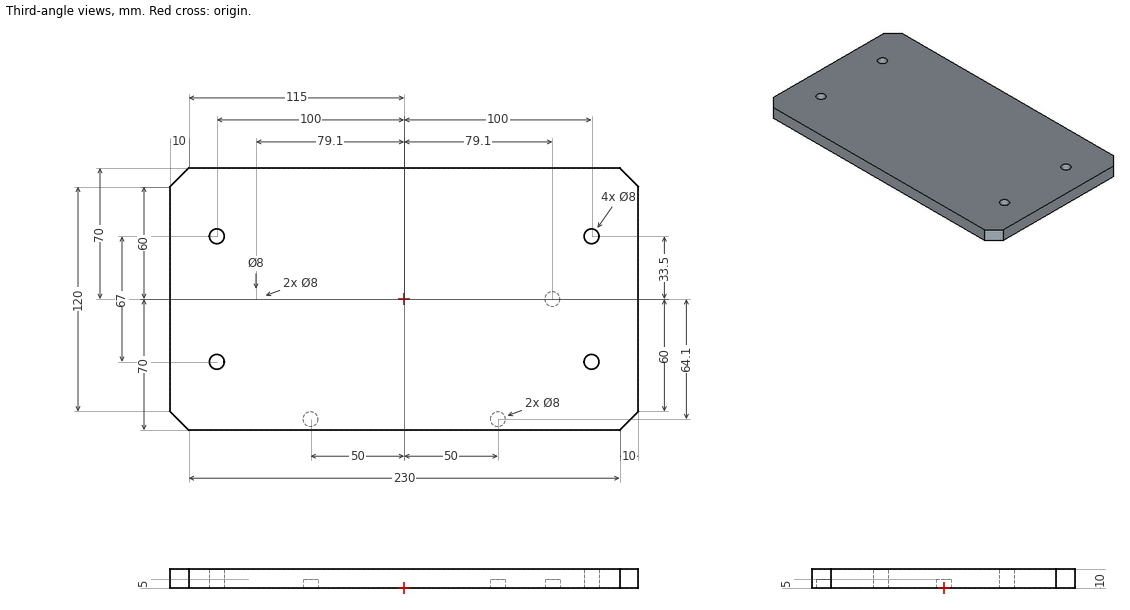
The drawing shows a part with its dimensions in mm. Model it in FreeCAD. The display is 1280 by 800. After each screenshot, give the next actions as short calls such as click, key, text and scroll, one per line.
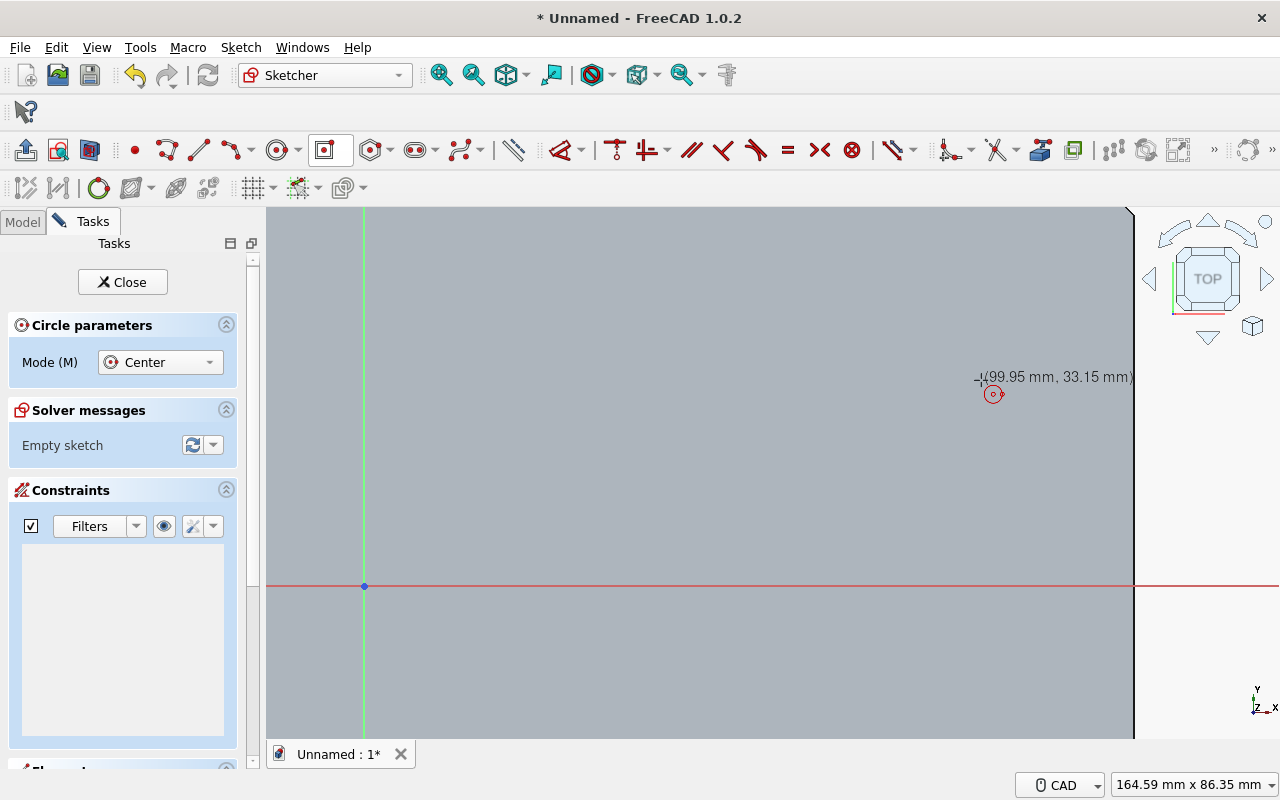
click(980, 380)
click(998, 362)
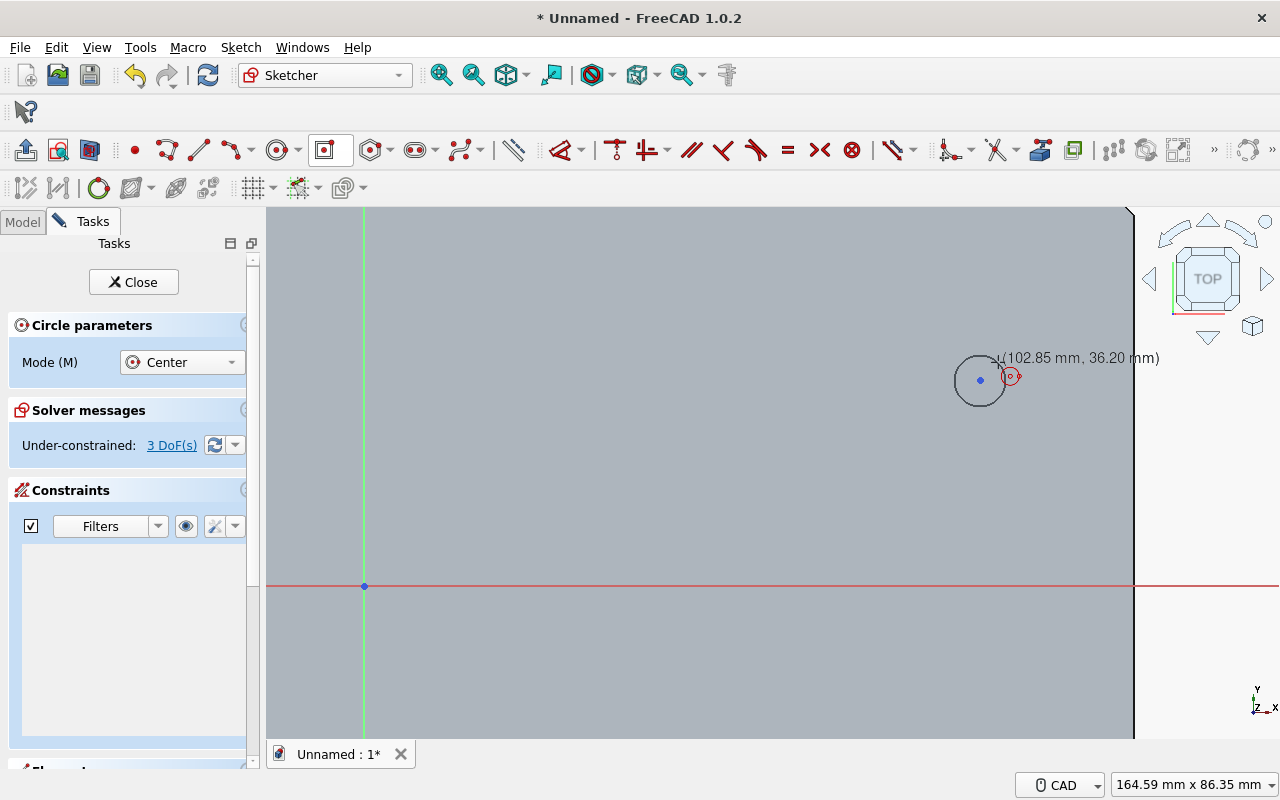
scroll(982, 381, down, 4)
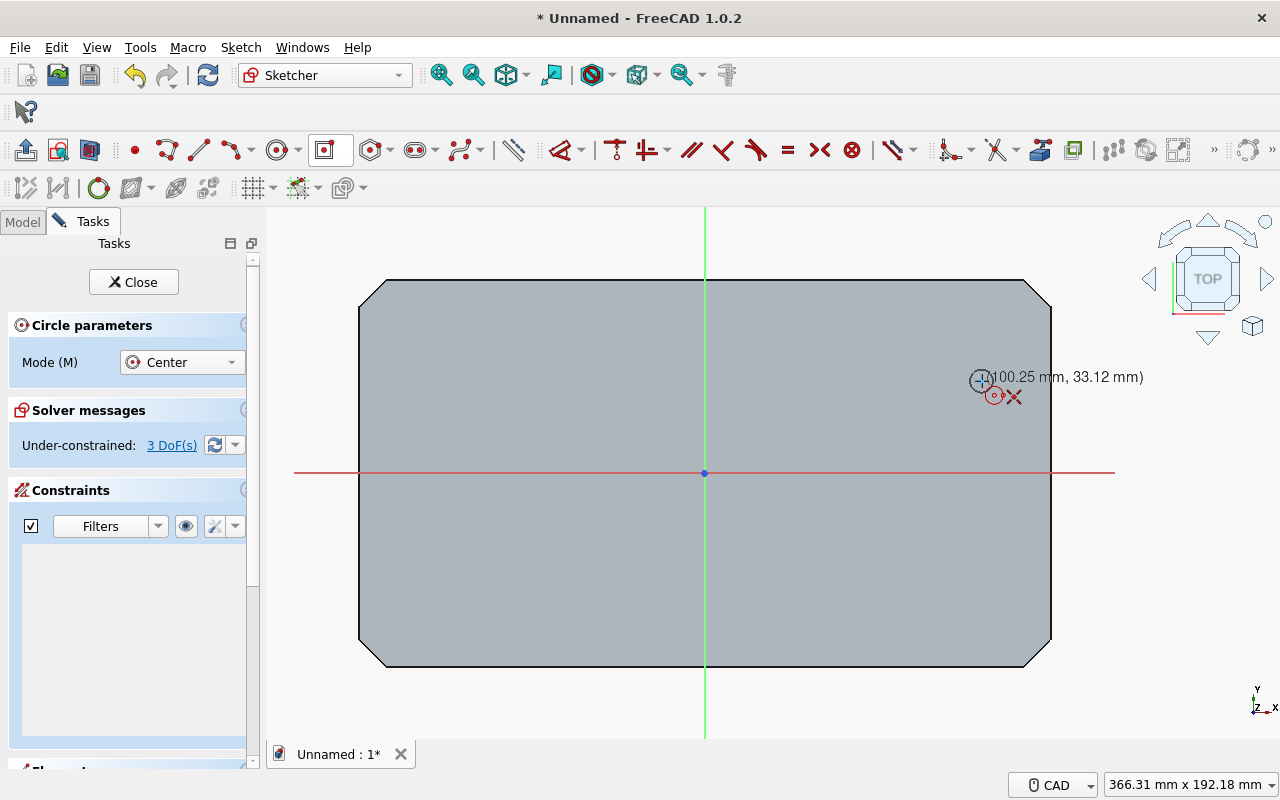
scroll(428, 381, up, 4)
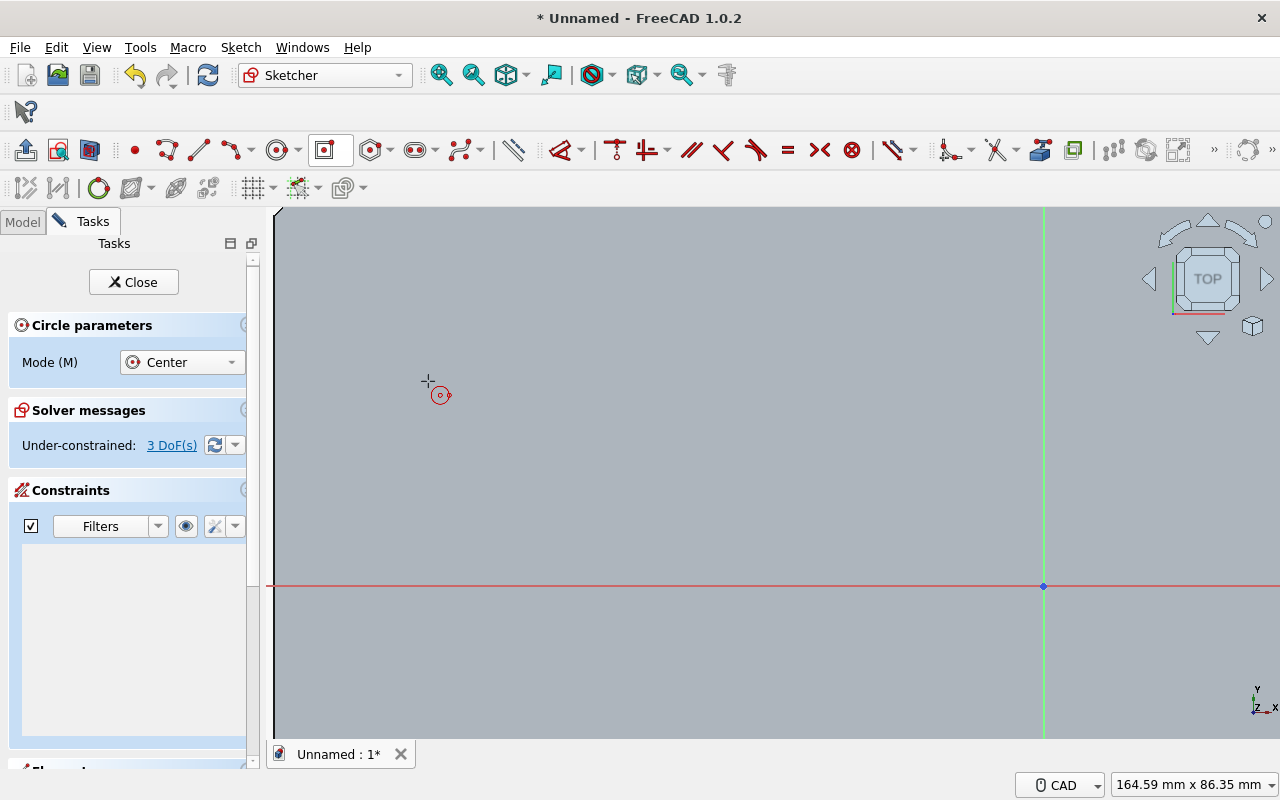
click(428, 380)
click(445, 362)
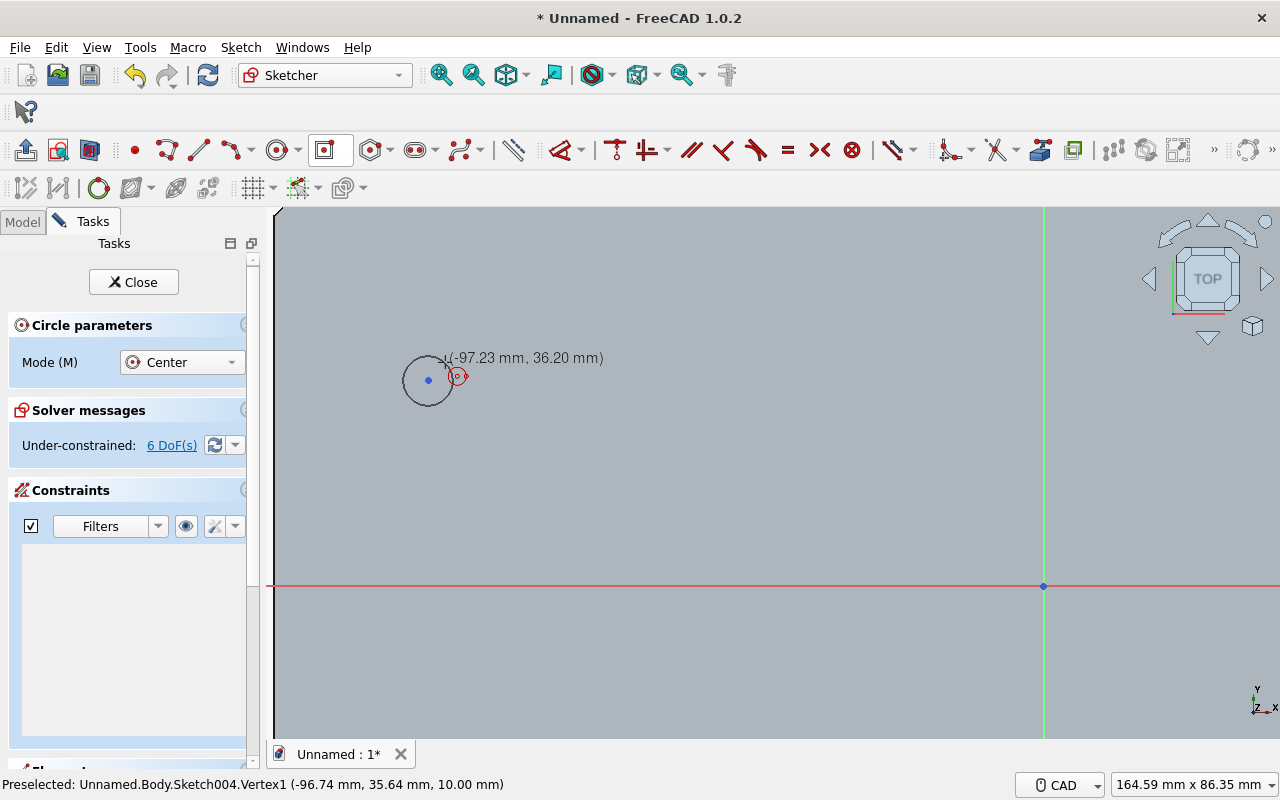
scroll(427, 381, down, 4)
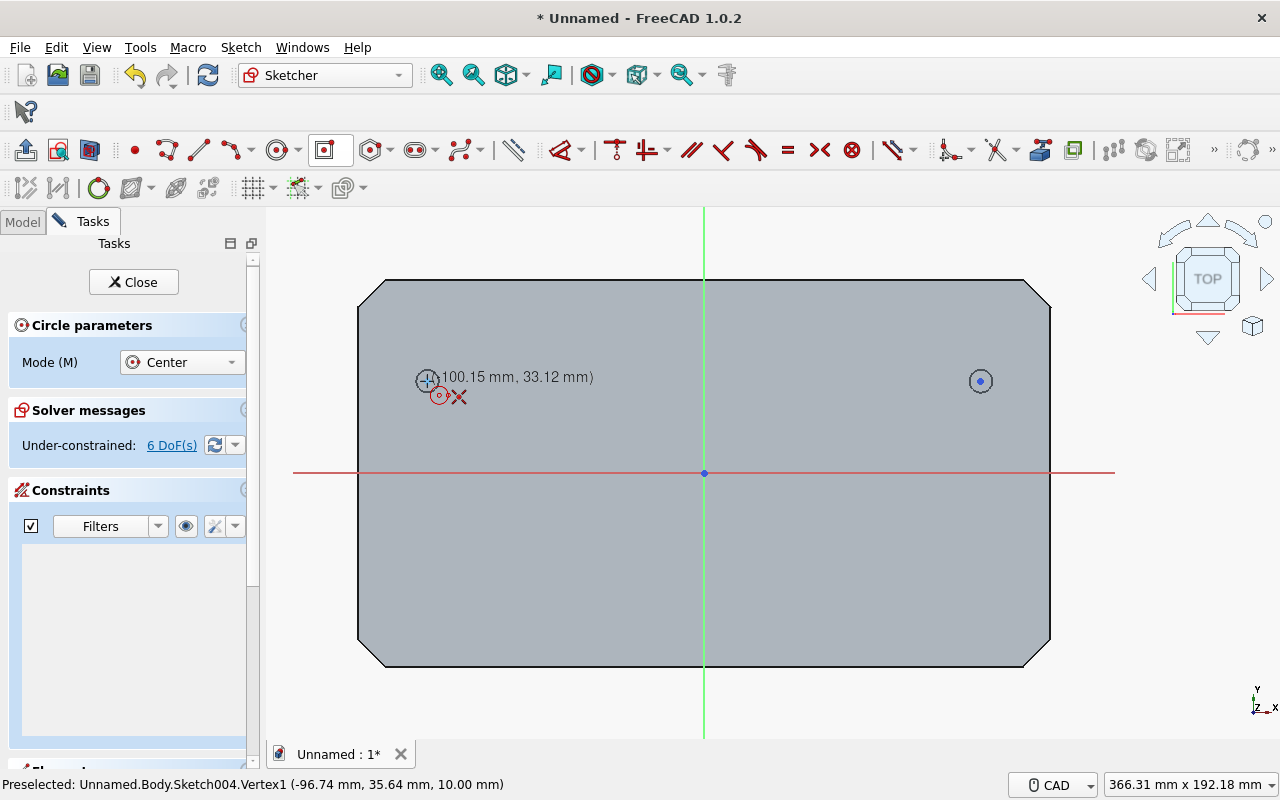
scroll(428, 566, up, 4)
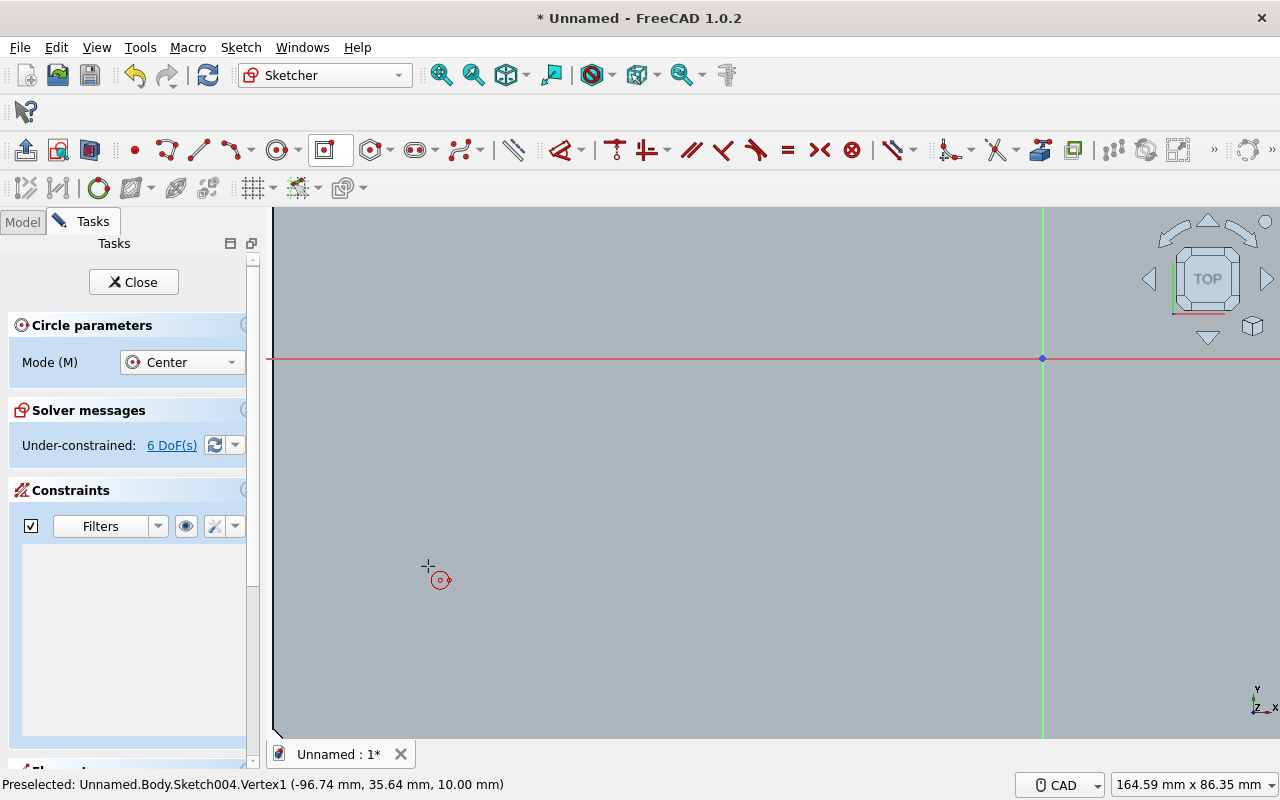
click(427, 565)
click(444, 548)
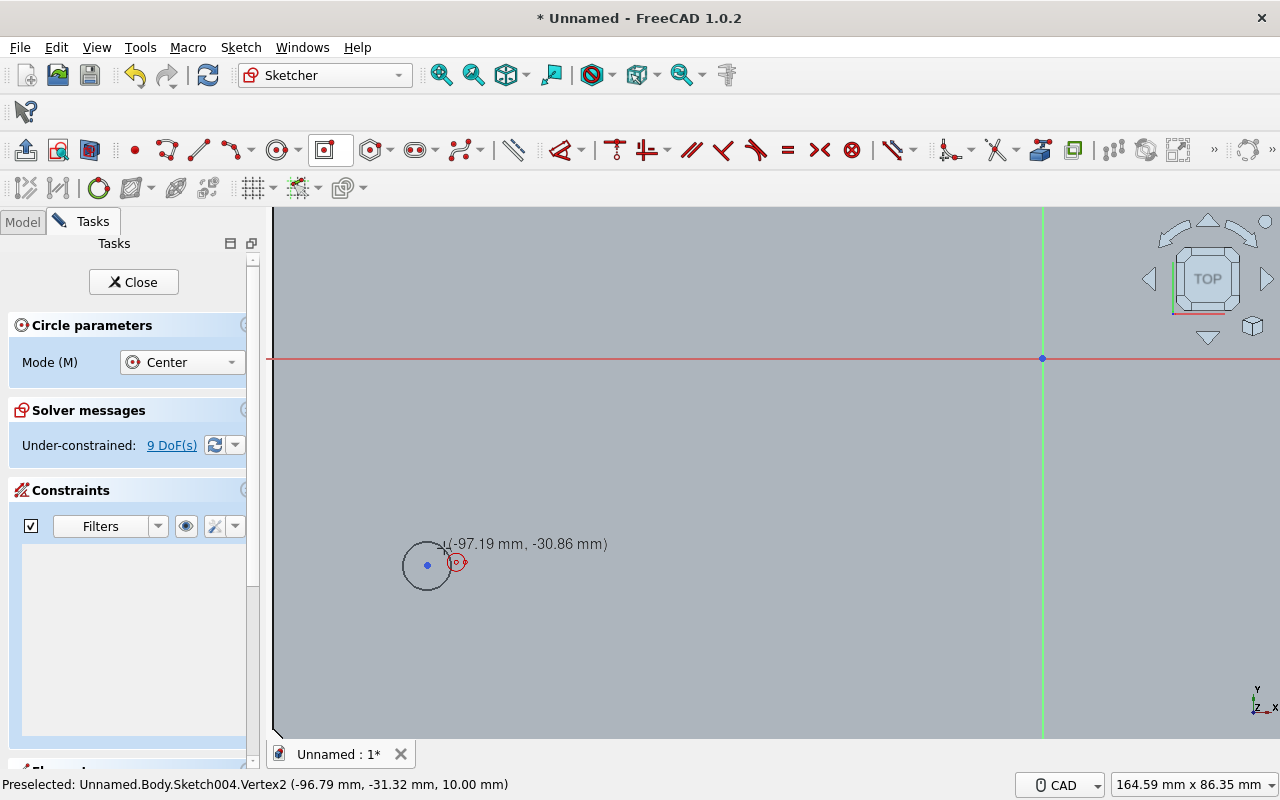
scroll(428, 566, down, 4)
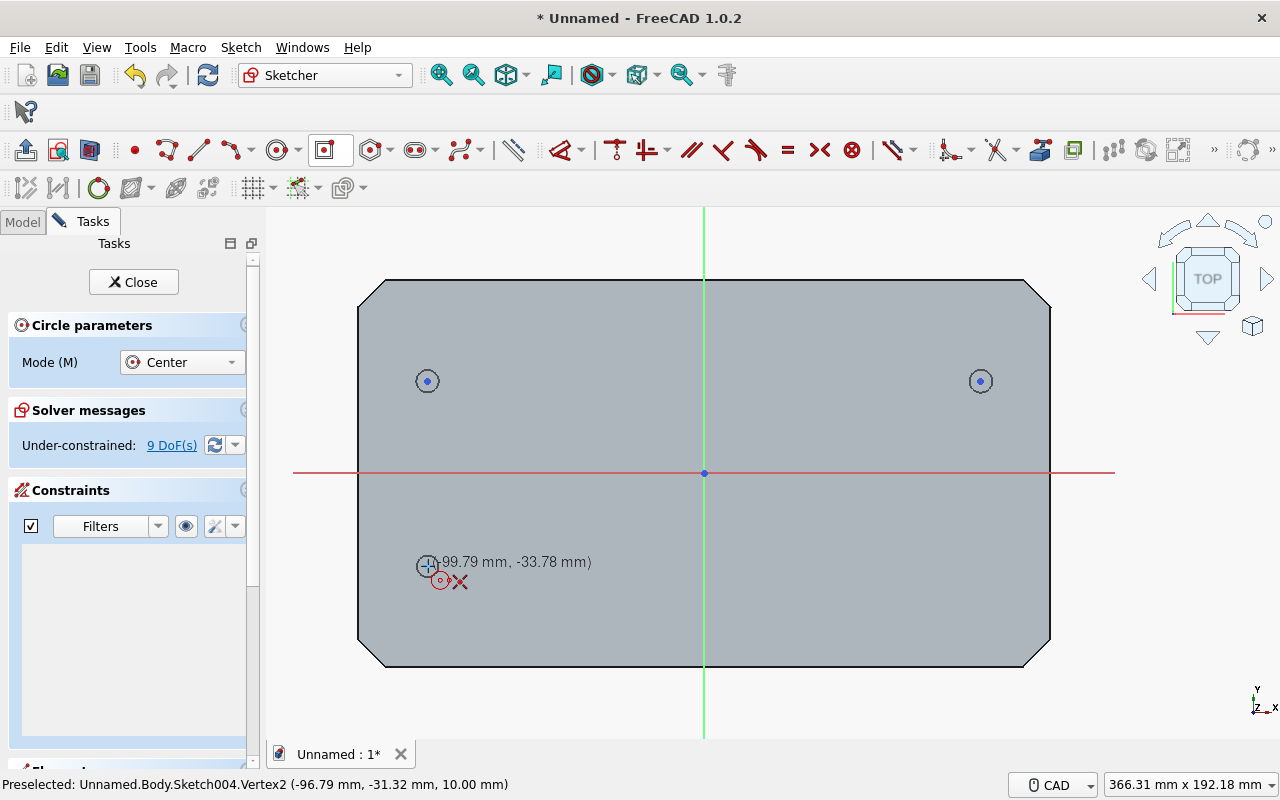
scroll(981, 566, up, 4)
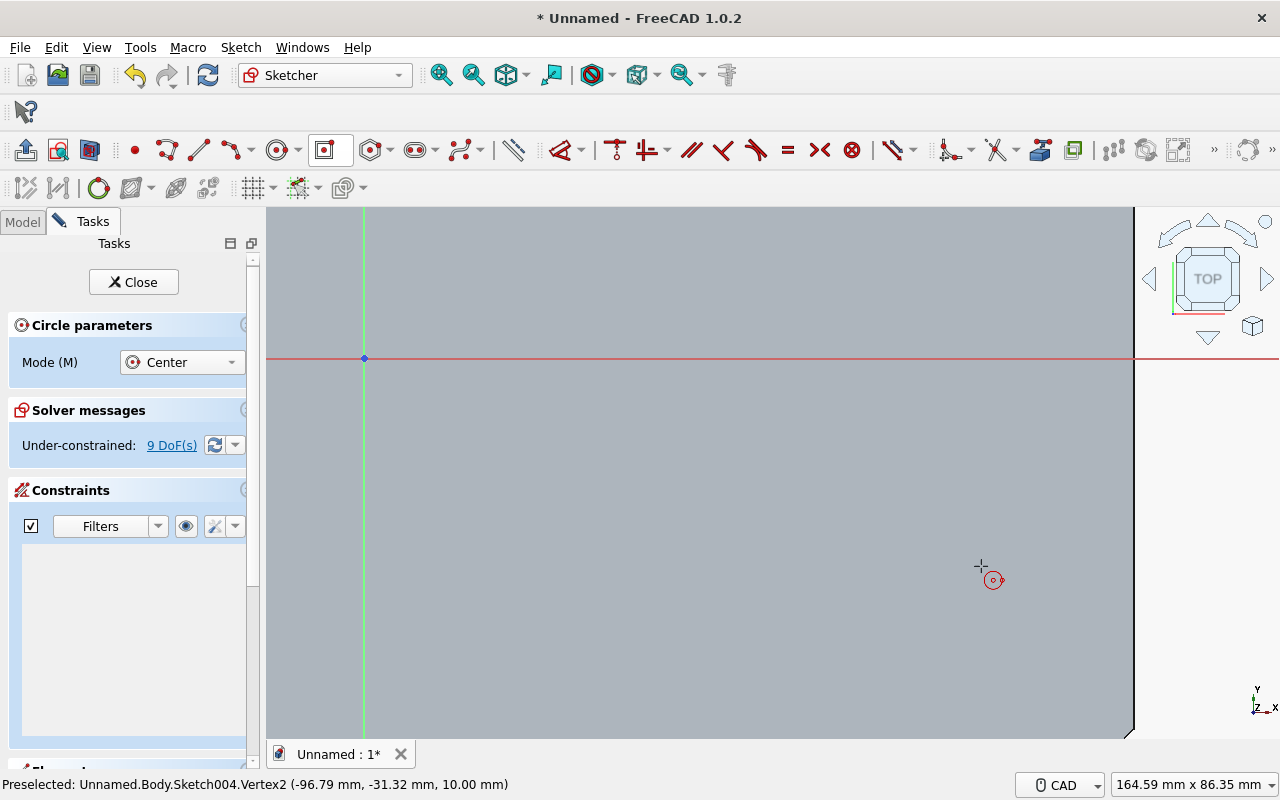
click(980, 565)
click(998, 548)
key(Escape)